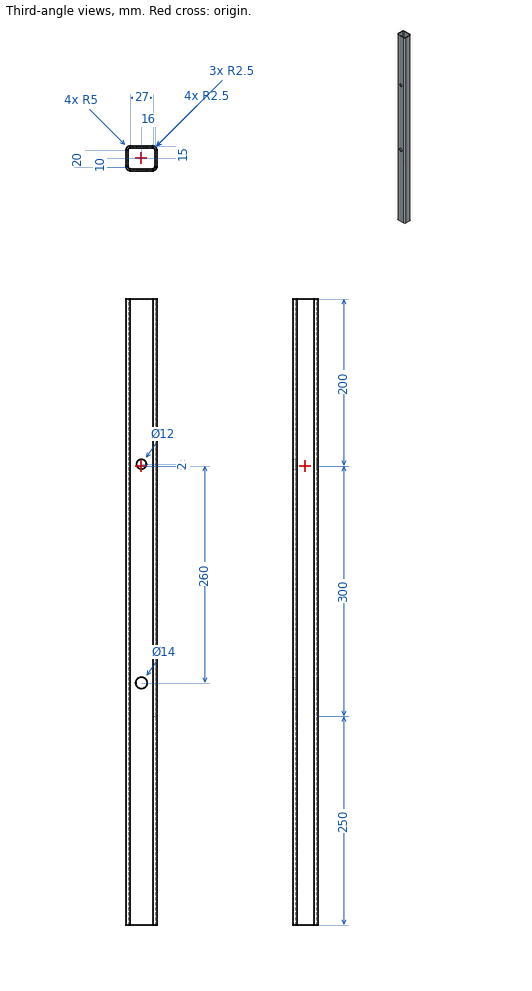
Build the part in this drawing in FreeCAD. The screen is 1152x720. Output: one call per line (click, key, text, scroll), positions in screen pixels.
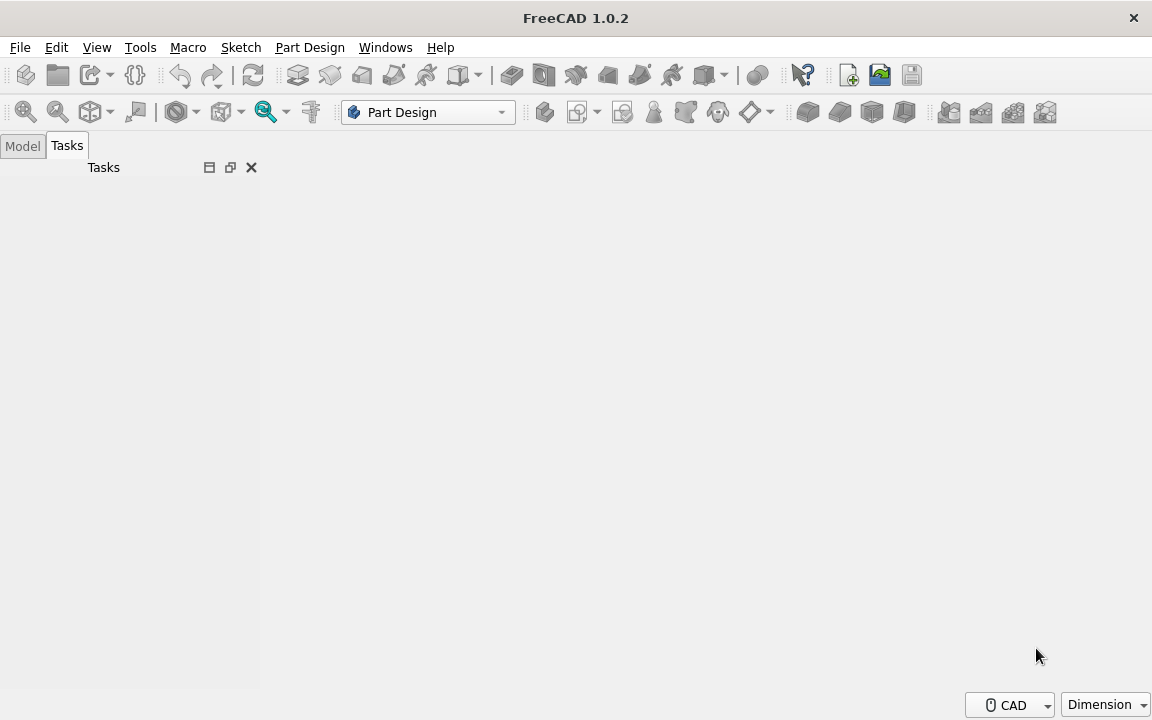
key(ctrl+n)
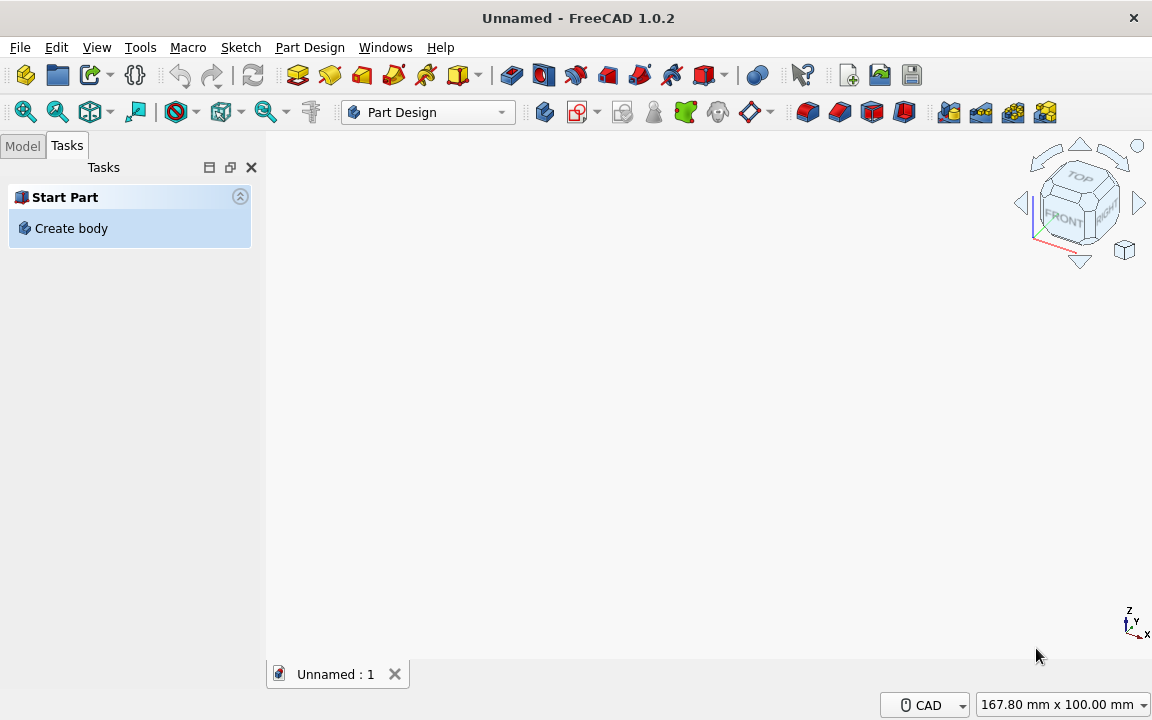
click(578, 112)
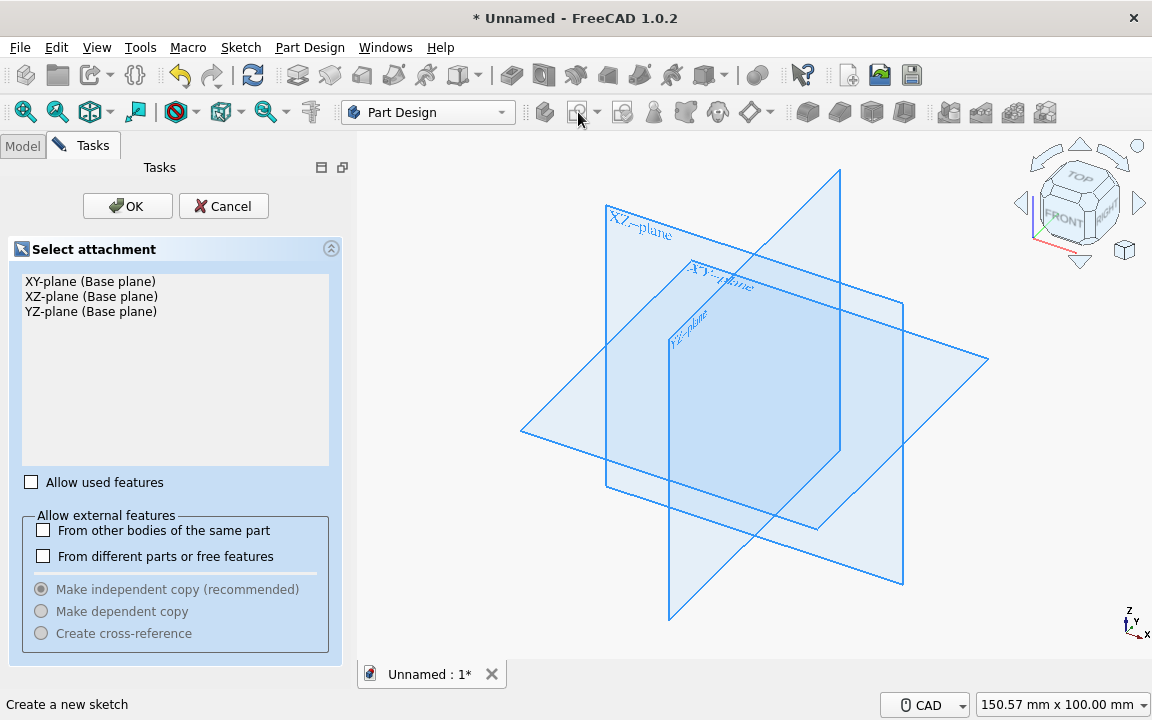
click(82, 282)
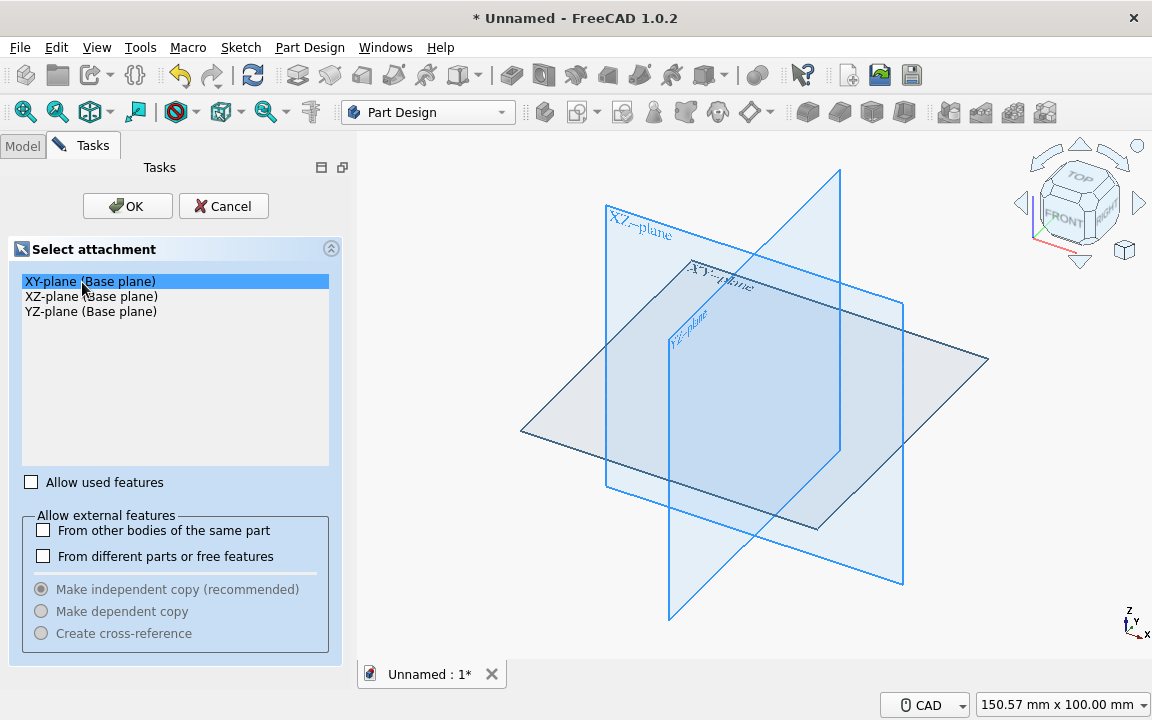
click(128, 206)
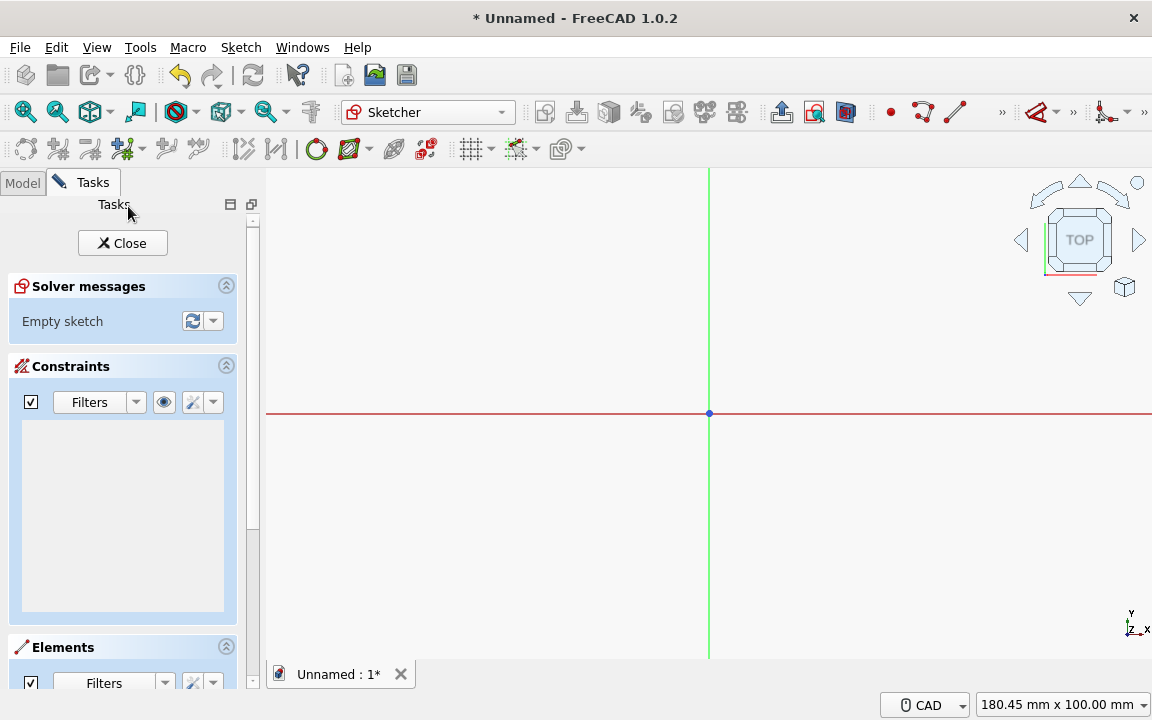
scroll(765, 413, up, 4)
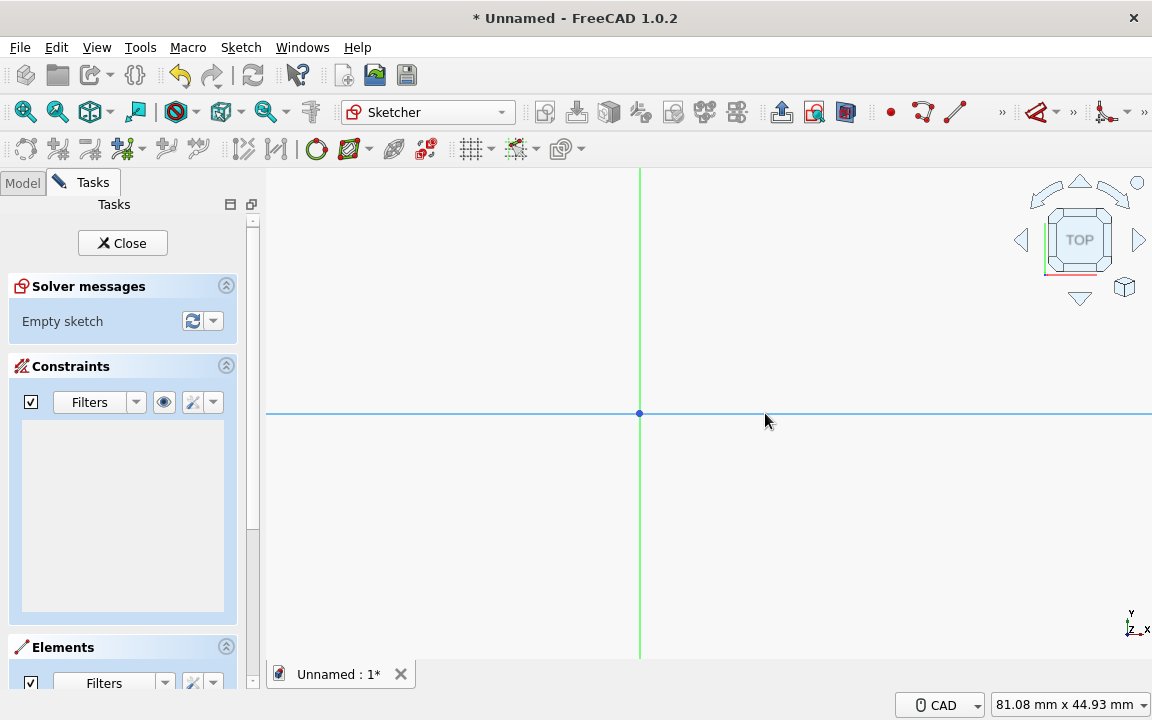
click(956, 112)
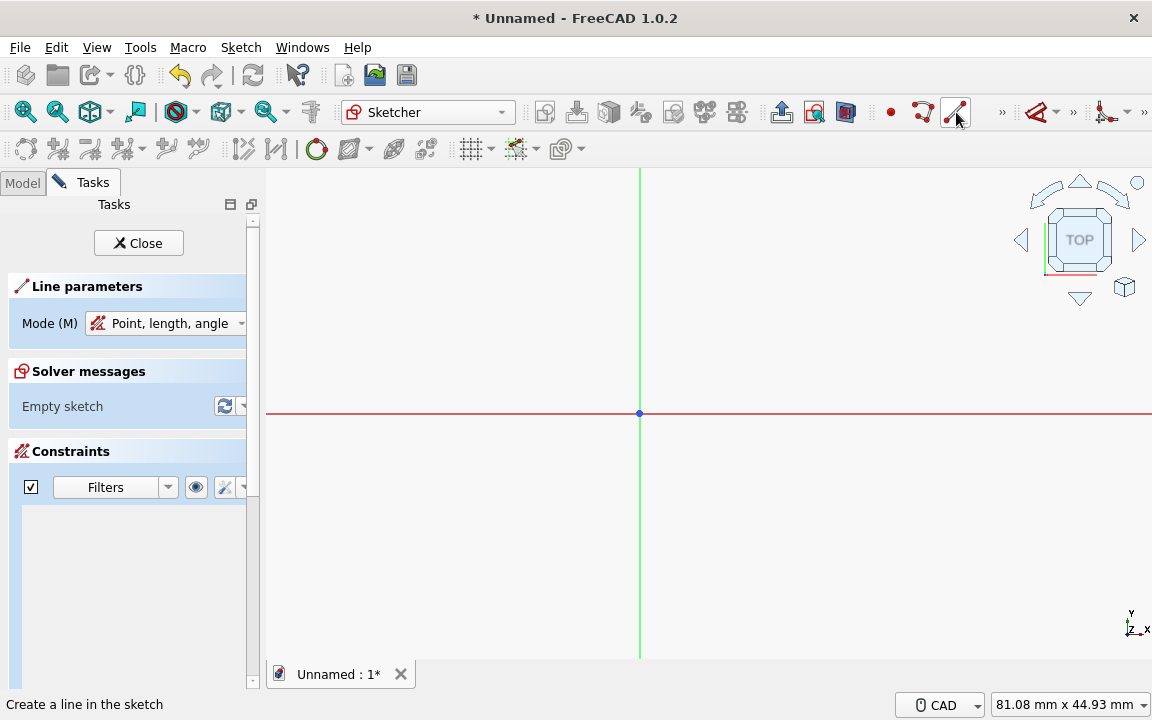
click(787, 250)
click(492, 250)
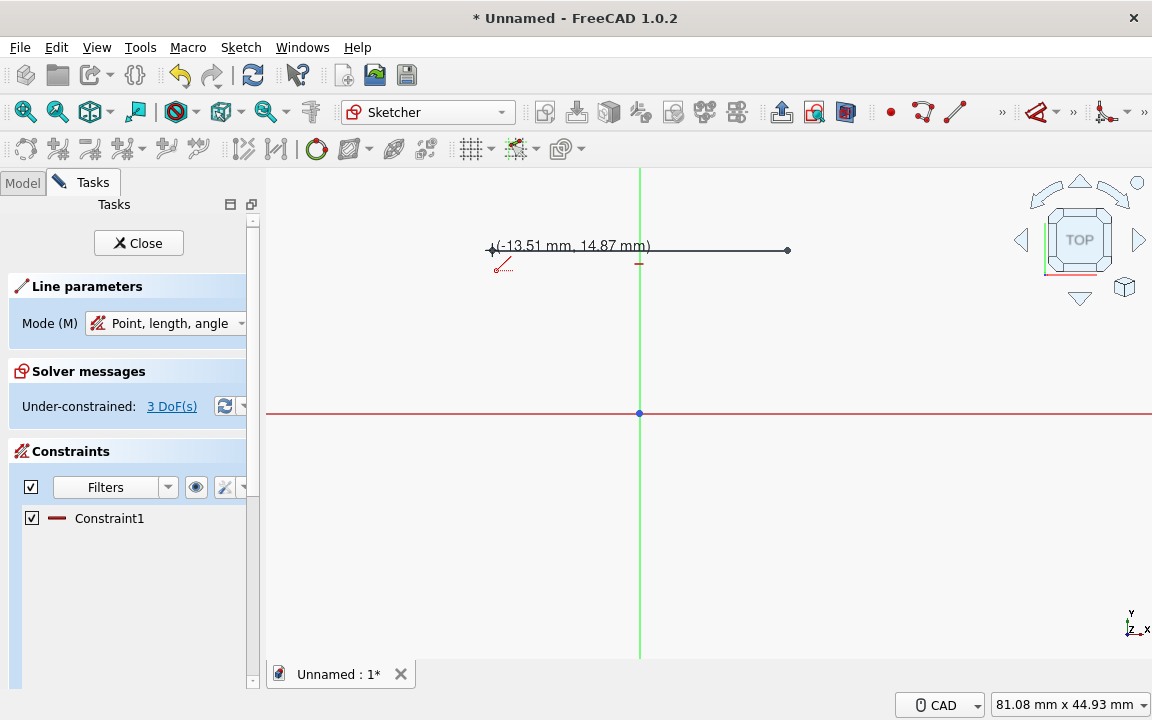
click(438, 304)
click(438, 523)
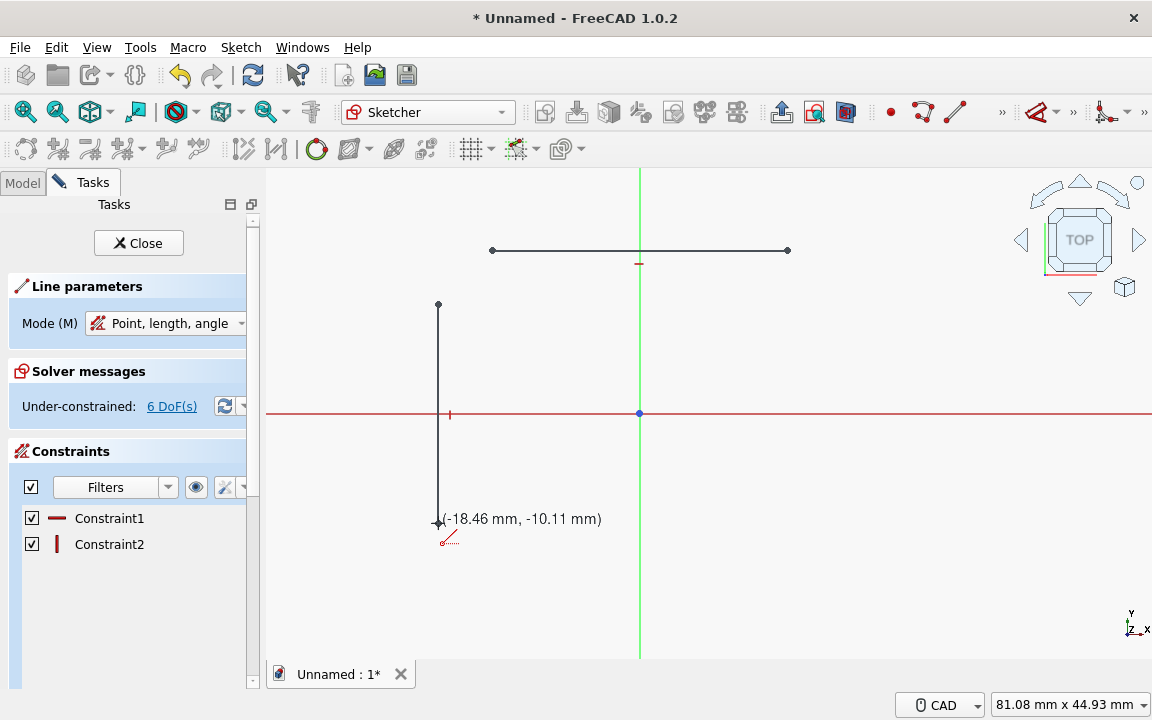
click(492, 577)
click(787, 577)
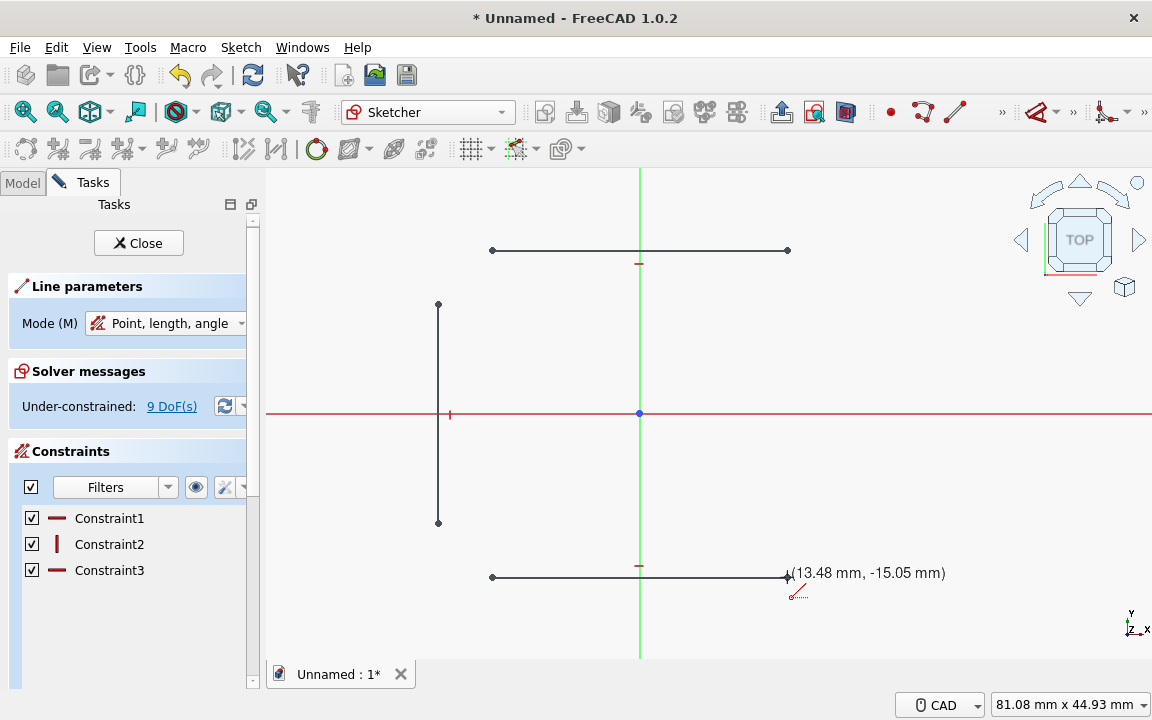
click(842, 523)
click(842, 304)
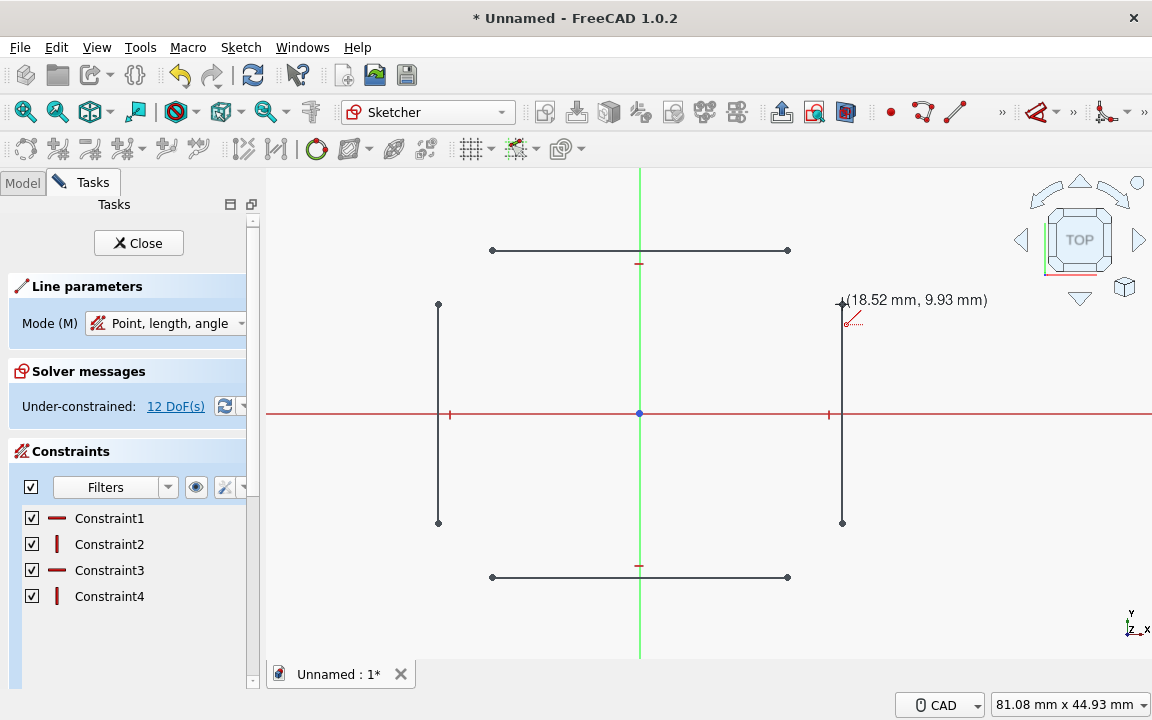
key(g)
key(3)
key(a)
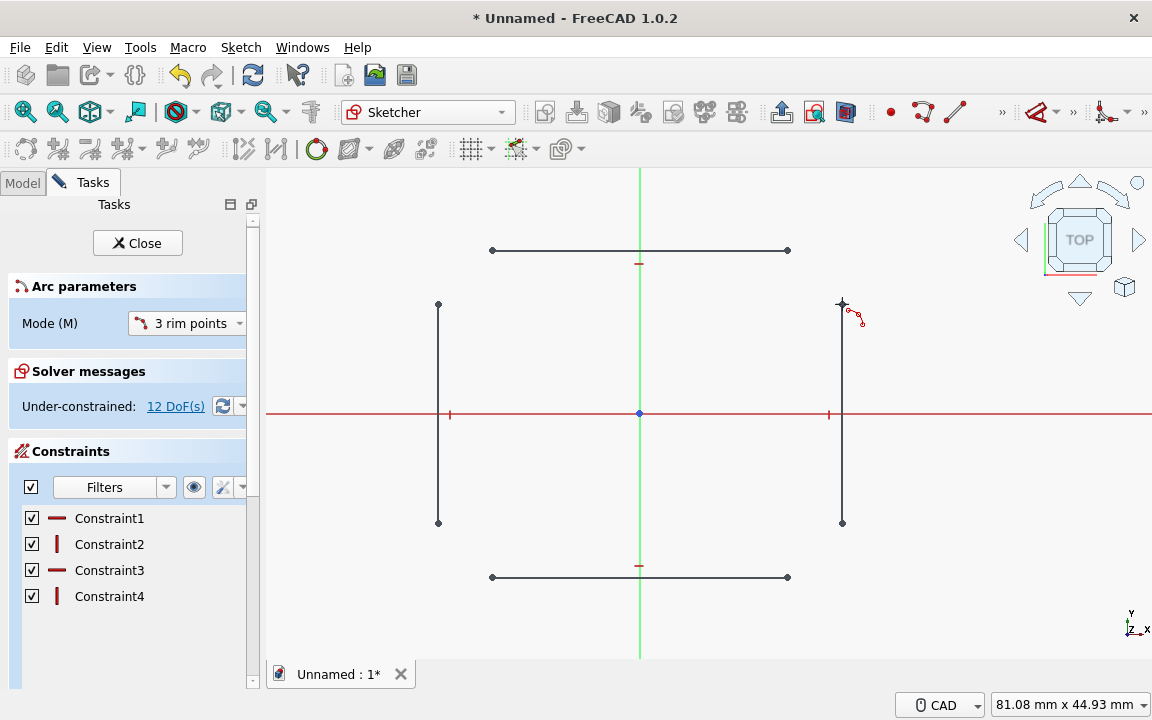
click(492, 251)
click(438, 305)
click(454, 266)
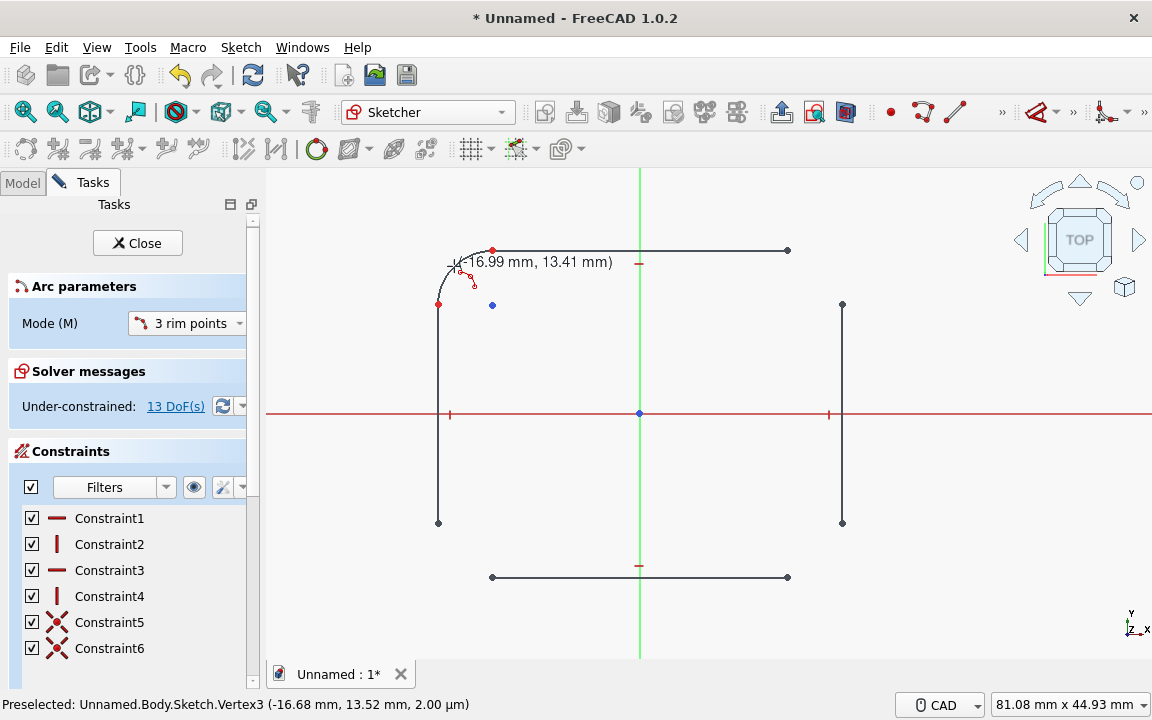
click(438, 524)
click(492, 578)
click(454, 561)